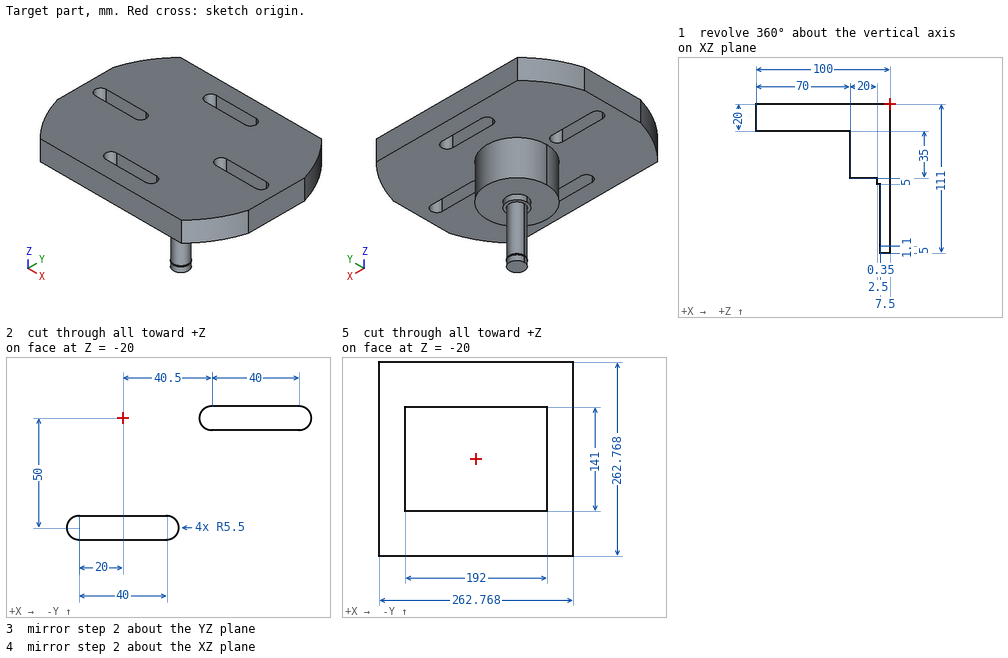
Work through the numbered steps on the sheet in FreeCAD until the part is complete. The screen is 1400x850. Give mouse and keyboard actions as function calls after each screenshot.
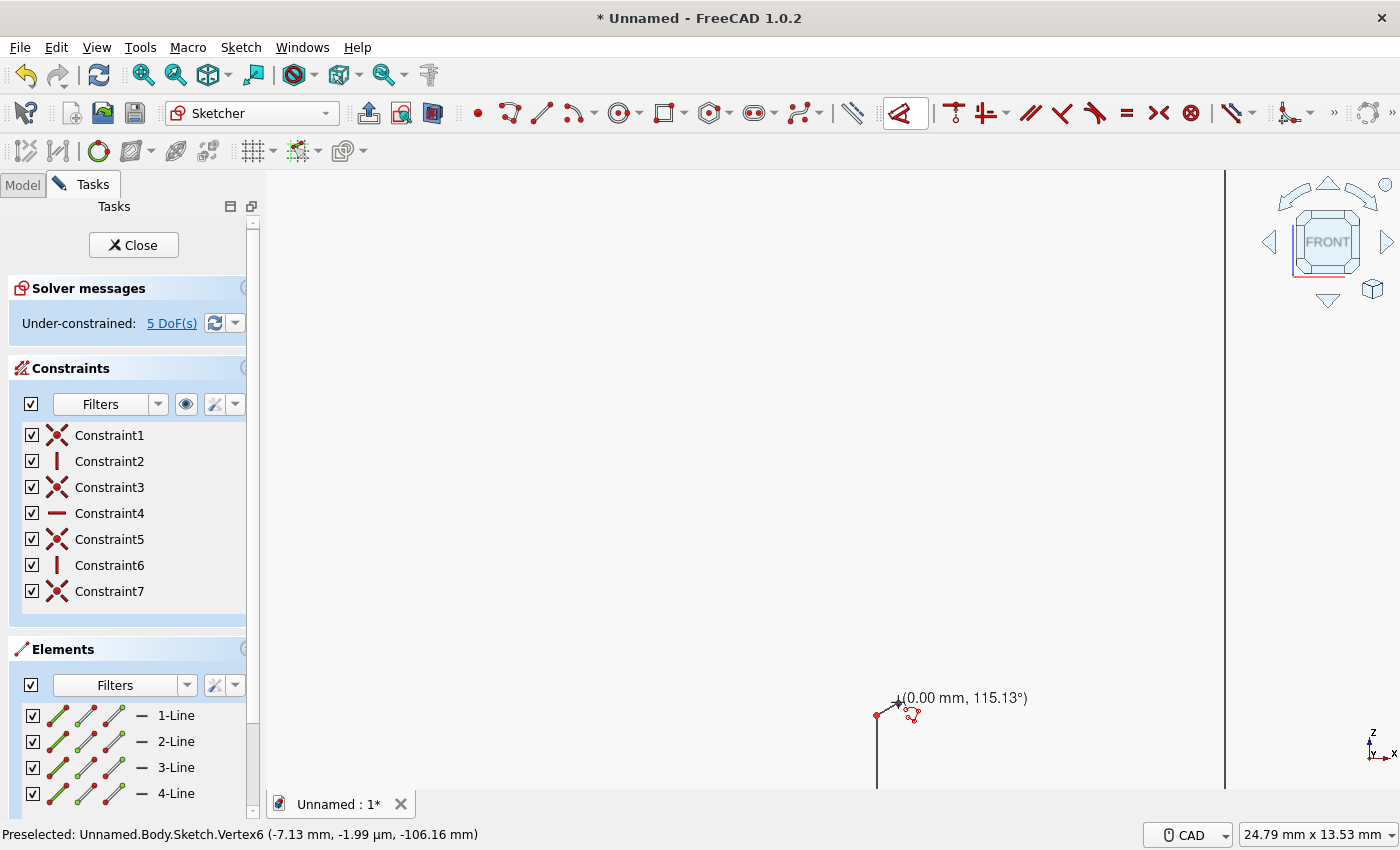
scroll(911, 647, down, 13)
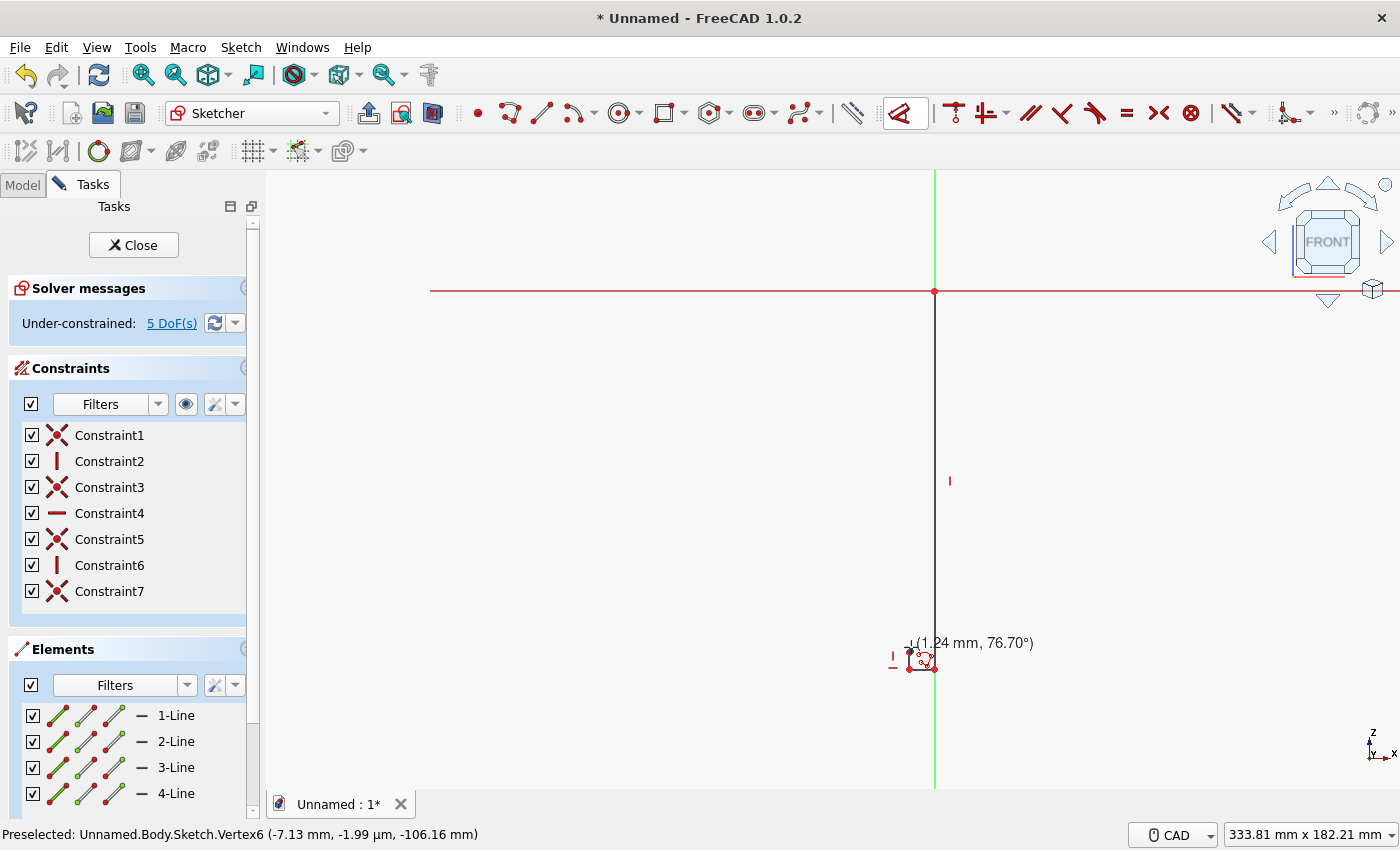
scroll(911, 648, up, 8)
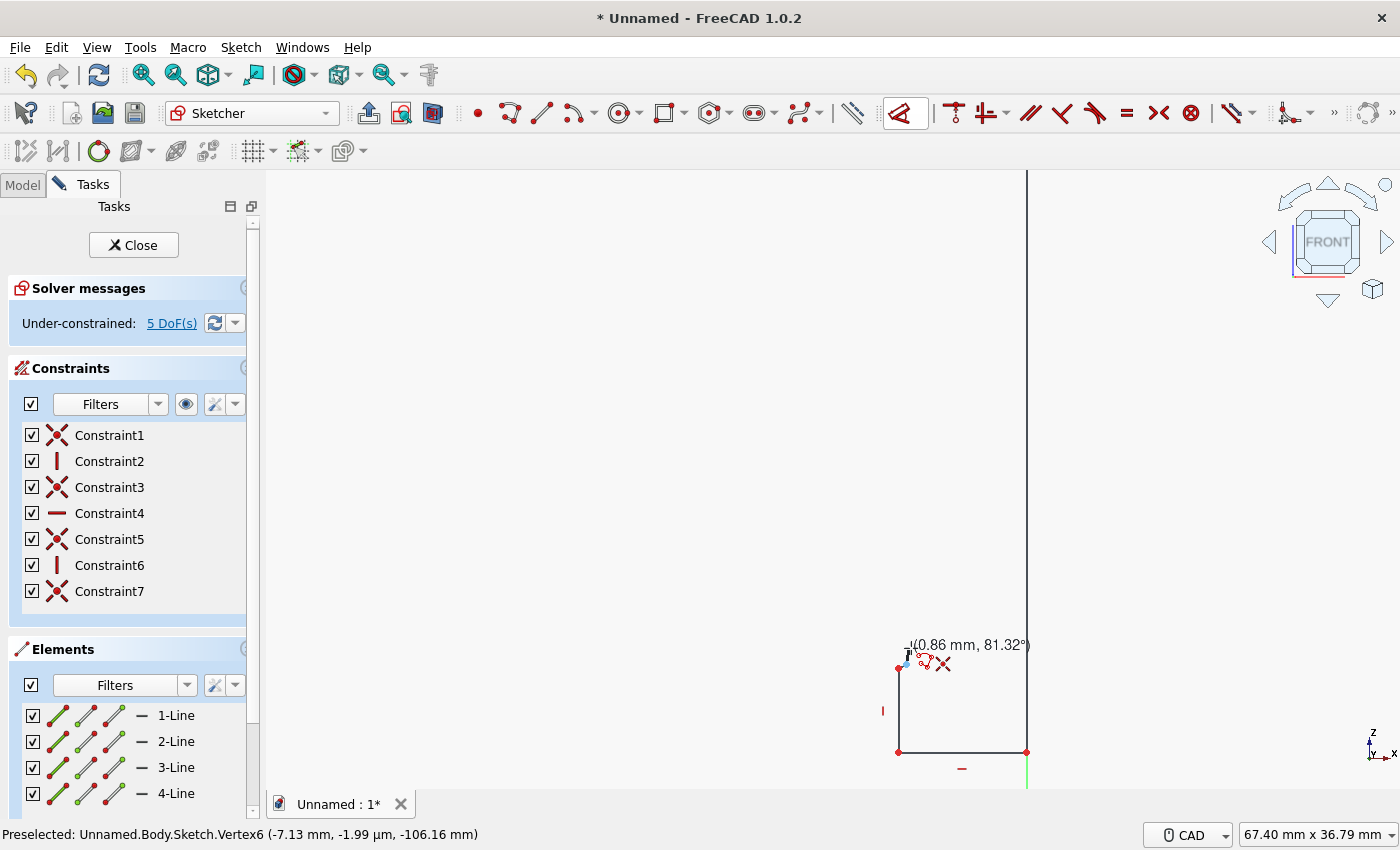
click(907, 643)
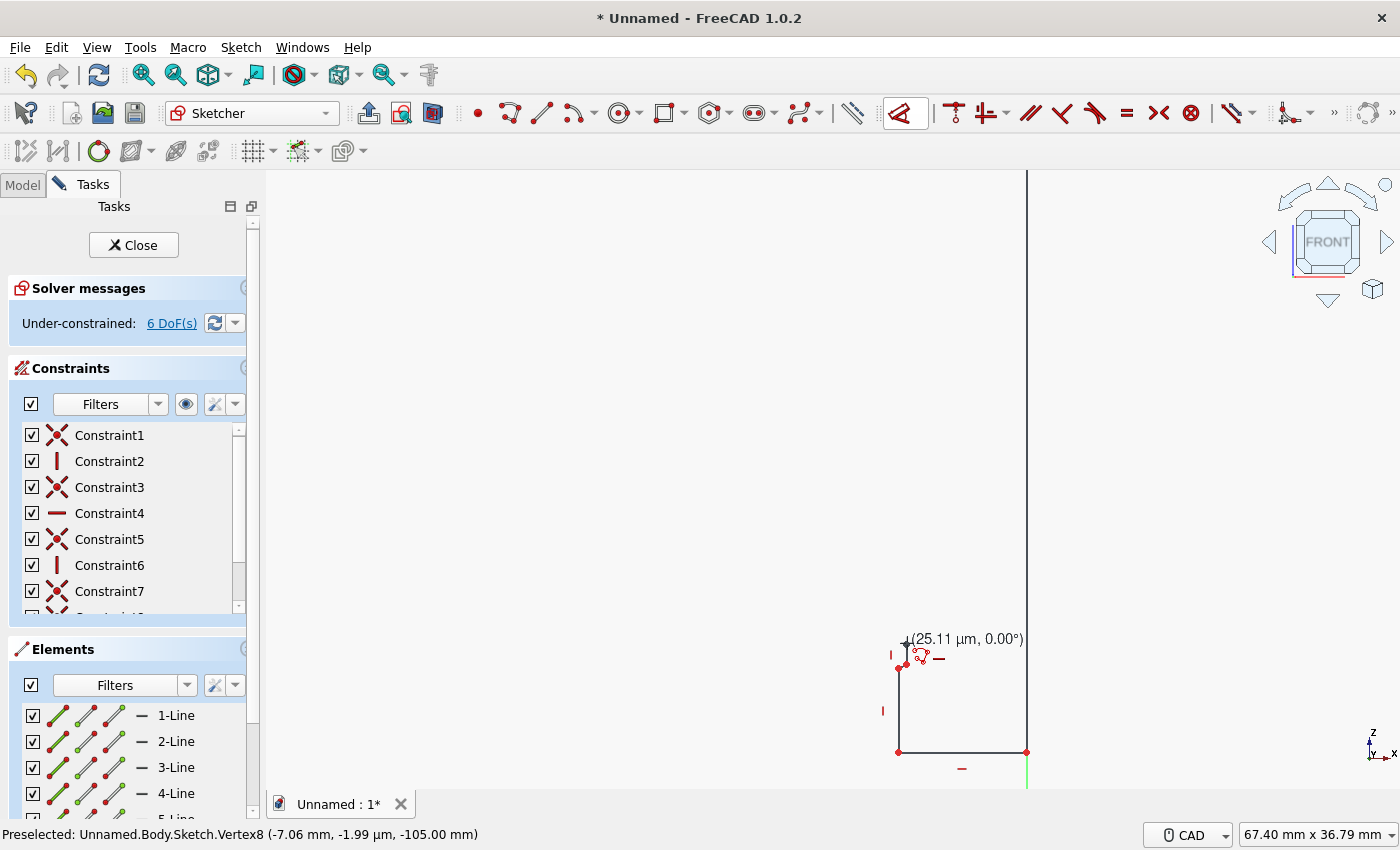
scroll(901, 643, up, 5)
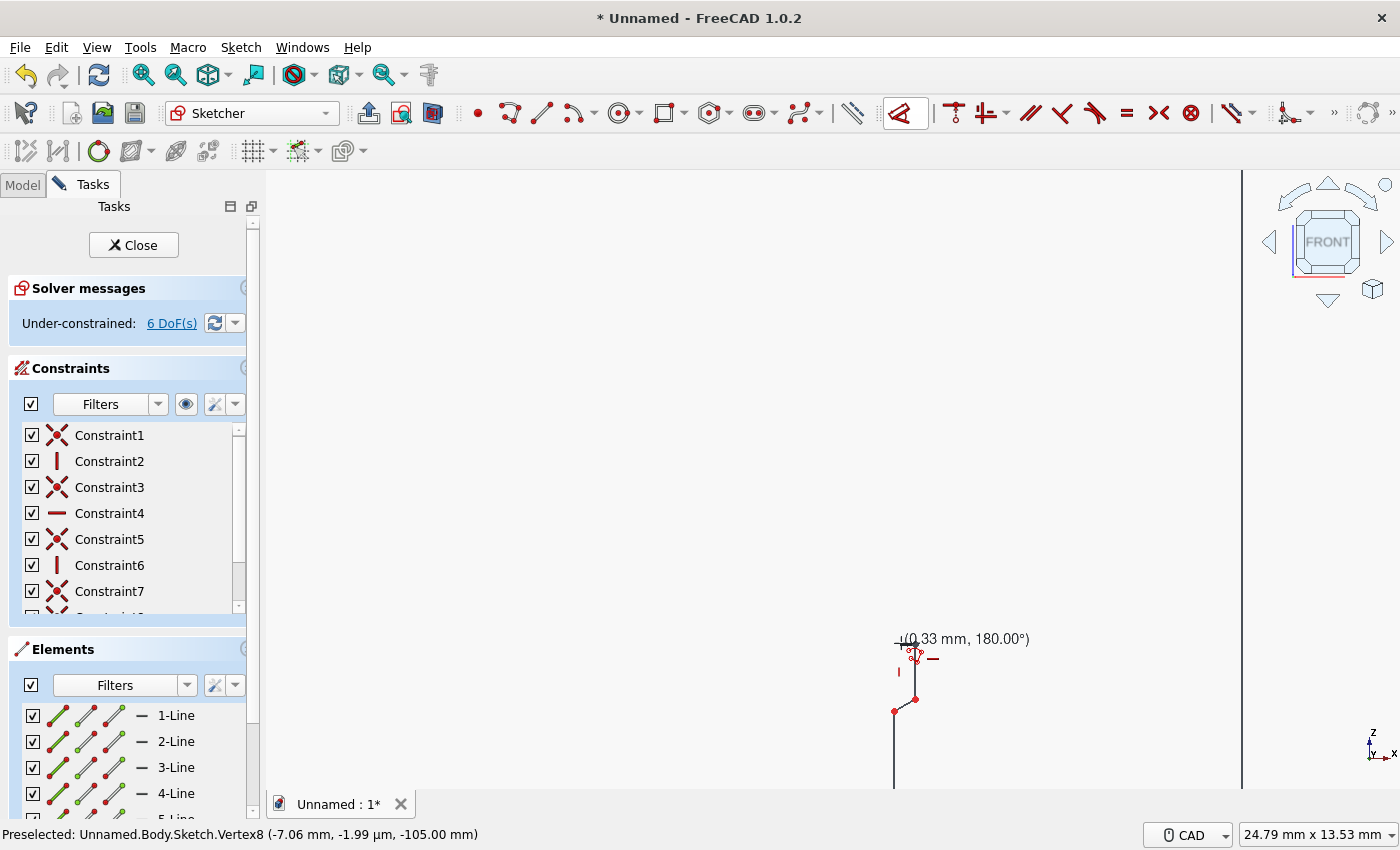
click(899, 642)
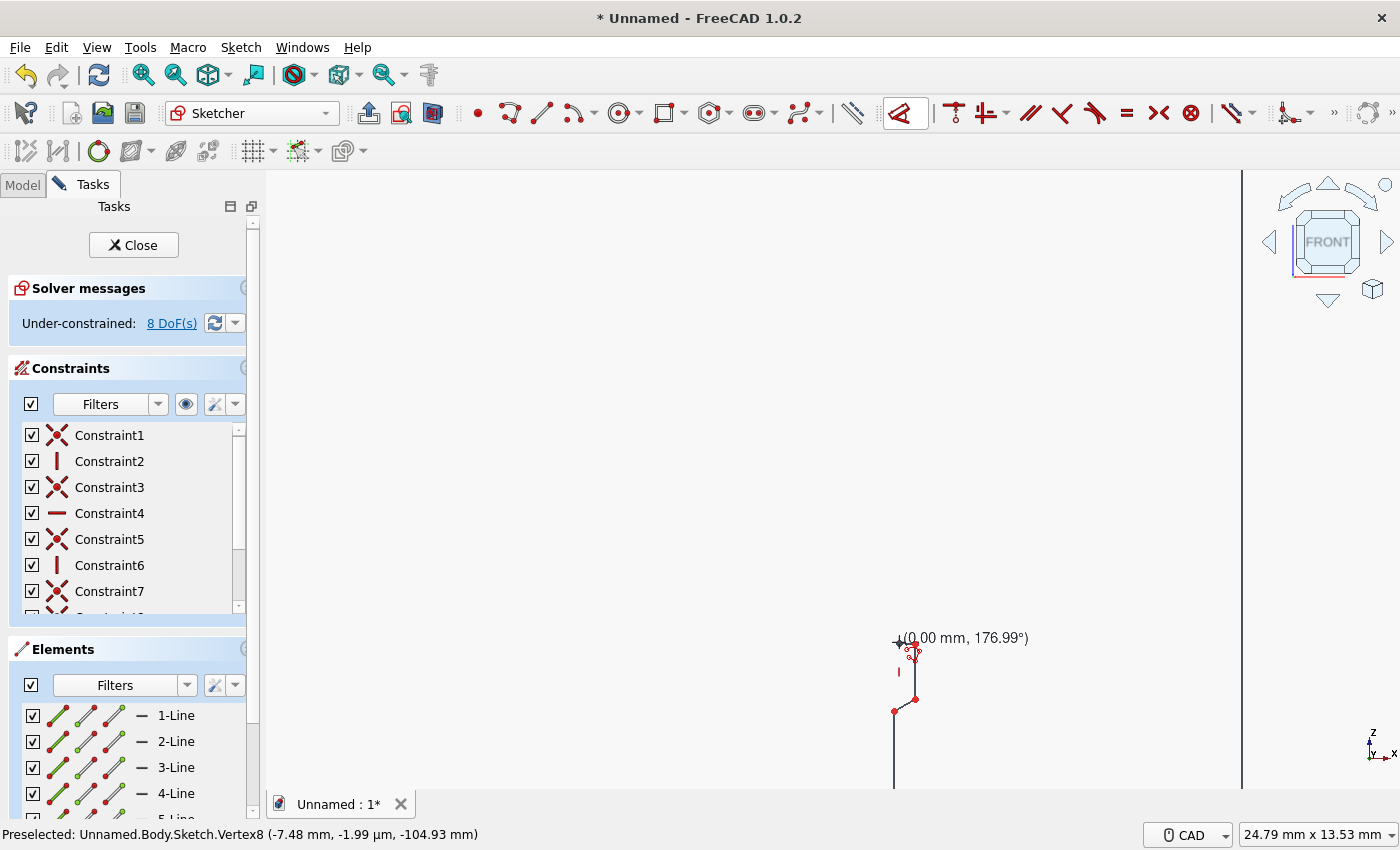
scroll(910, 648, down, 13)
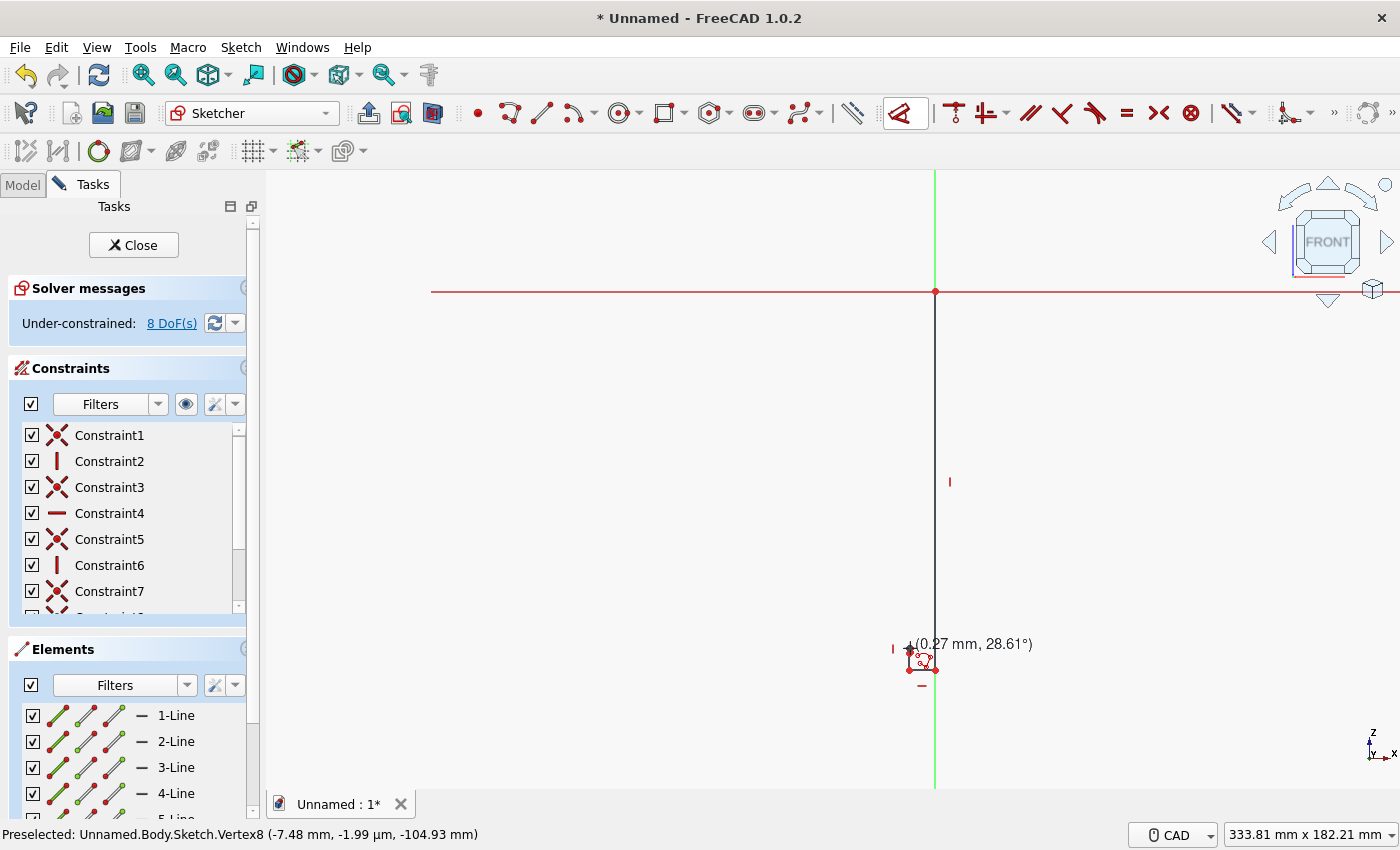
click(910, 496)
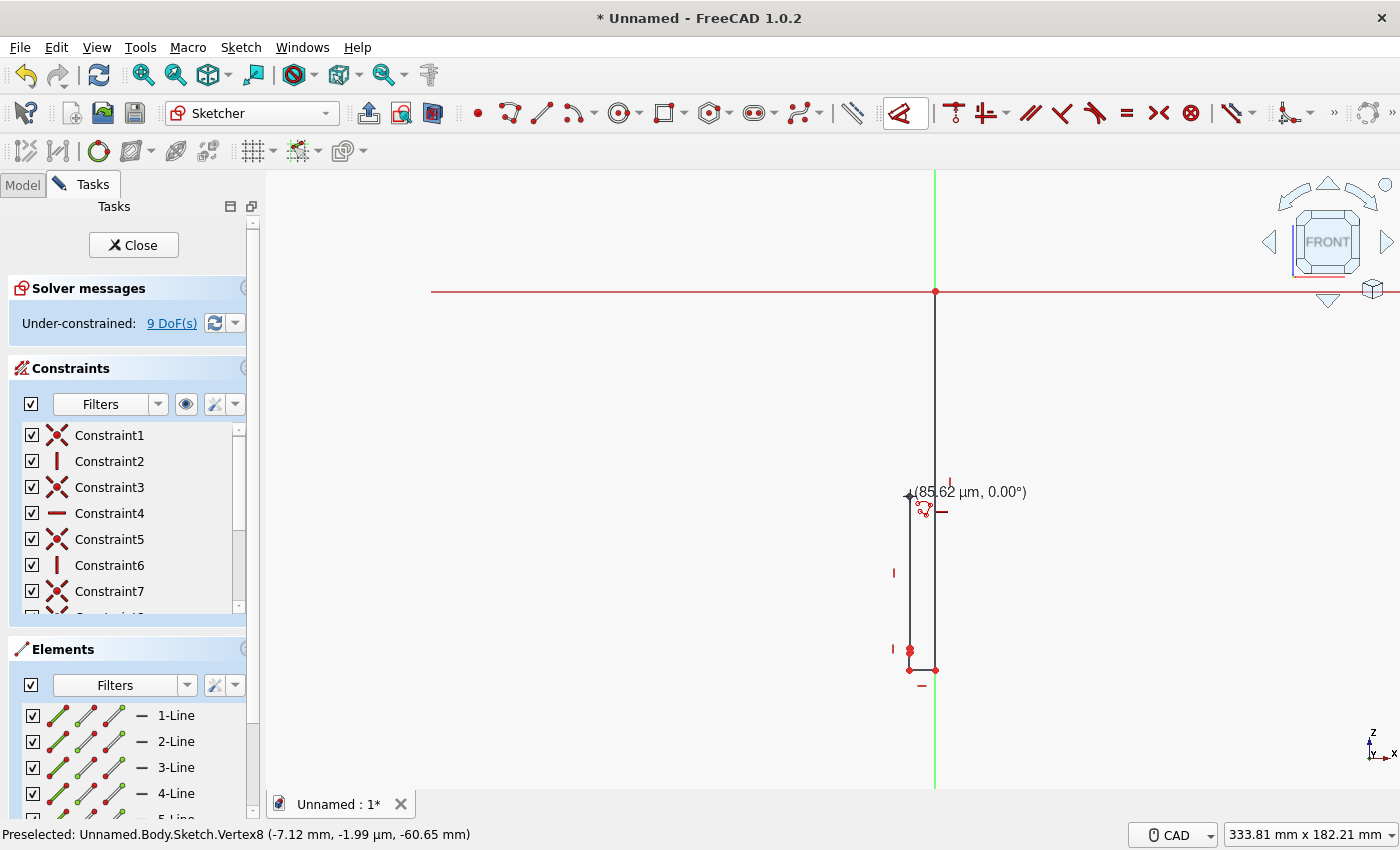
scroll(901, 496, up, 4)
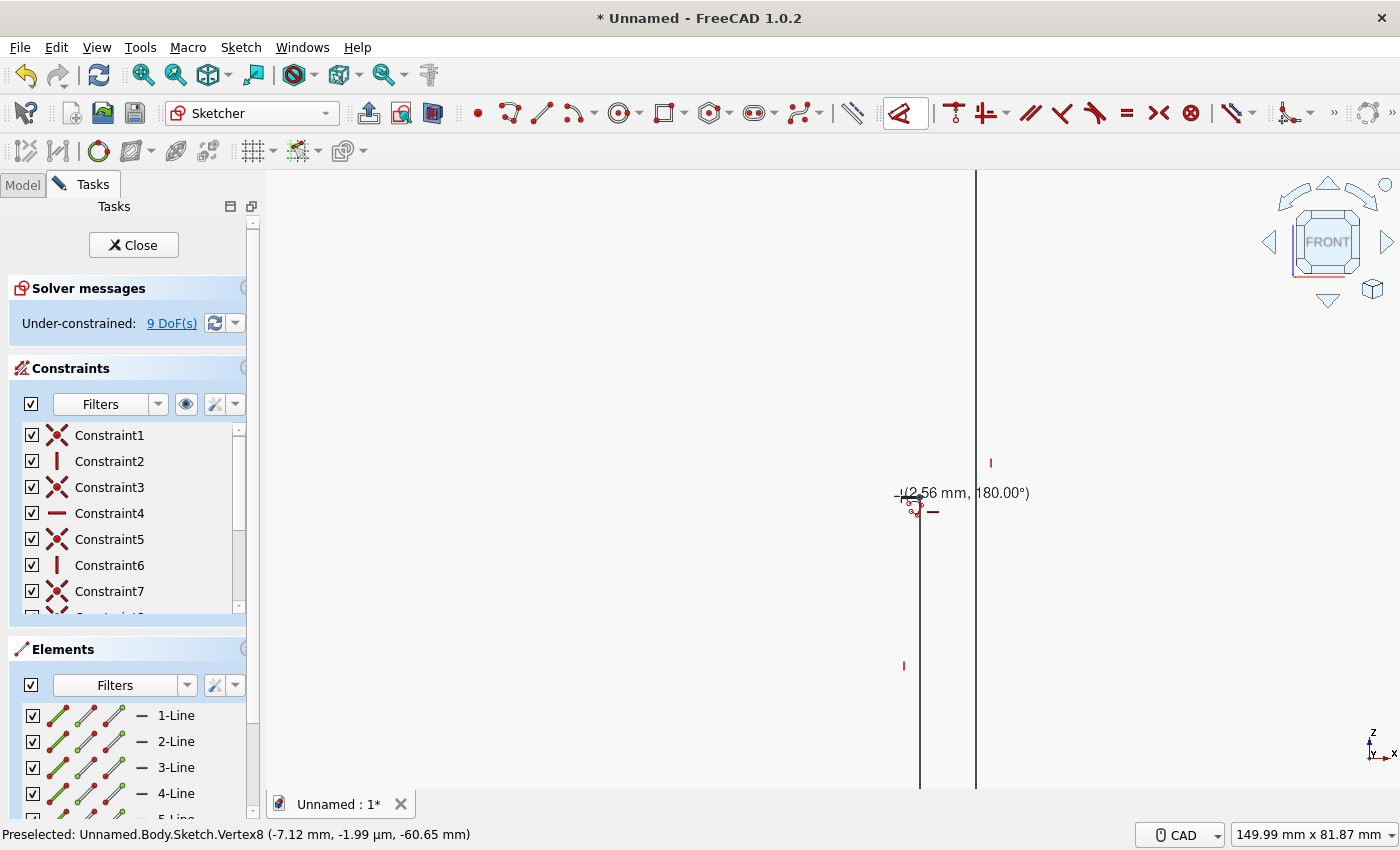
click(901, 495)
click(901, 457)
click(750, 457)